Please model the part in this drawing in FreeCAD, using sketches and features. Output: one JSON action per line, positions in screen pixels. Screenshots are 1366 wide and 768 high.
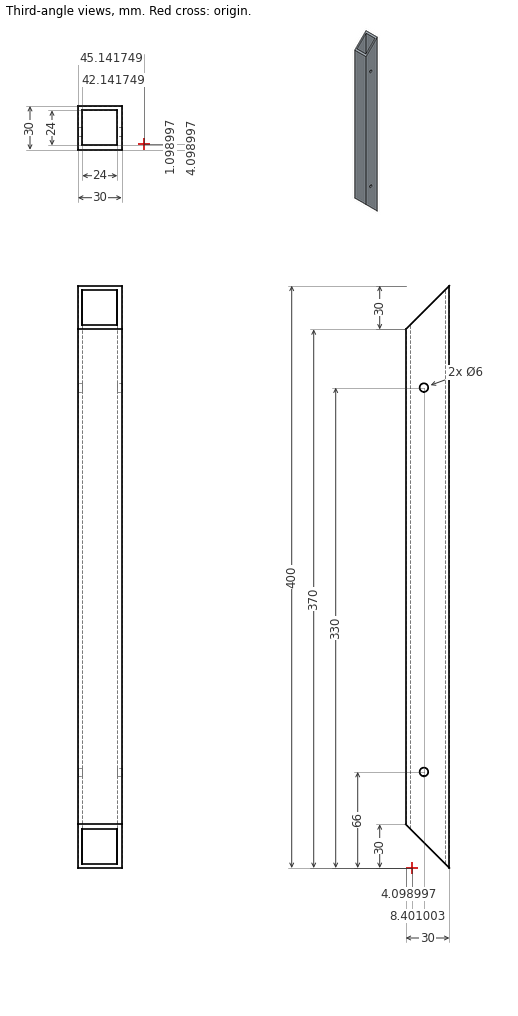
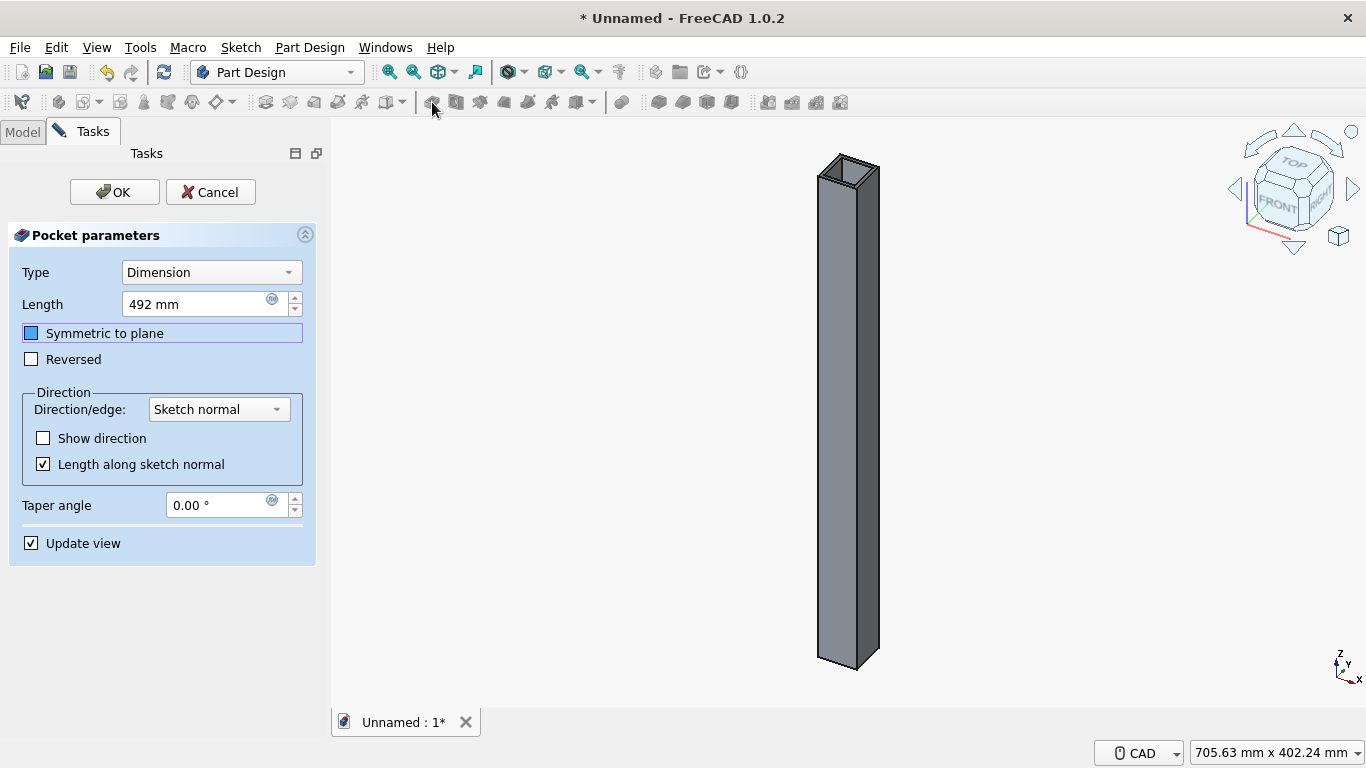
{"action": "left_click", "coordinate": [115, 192]}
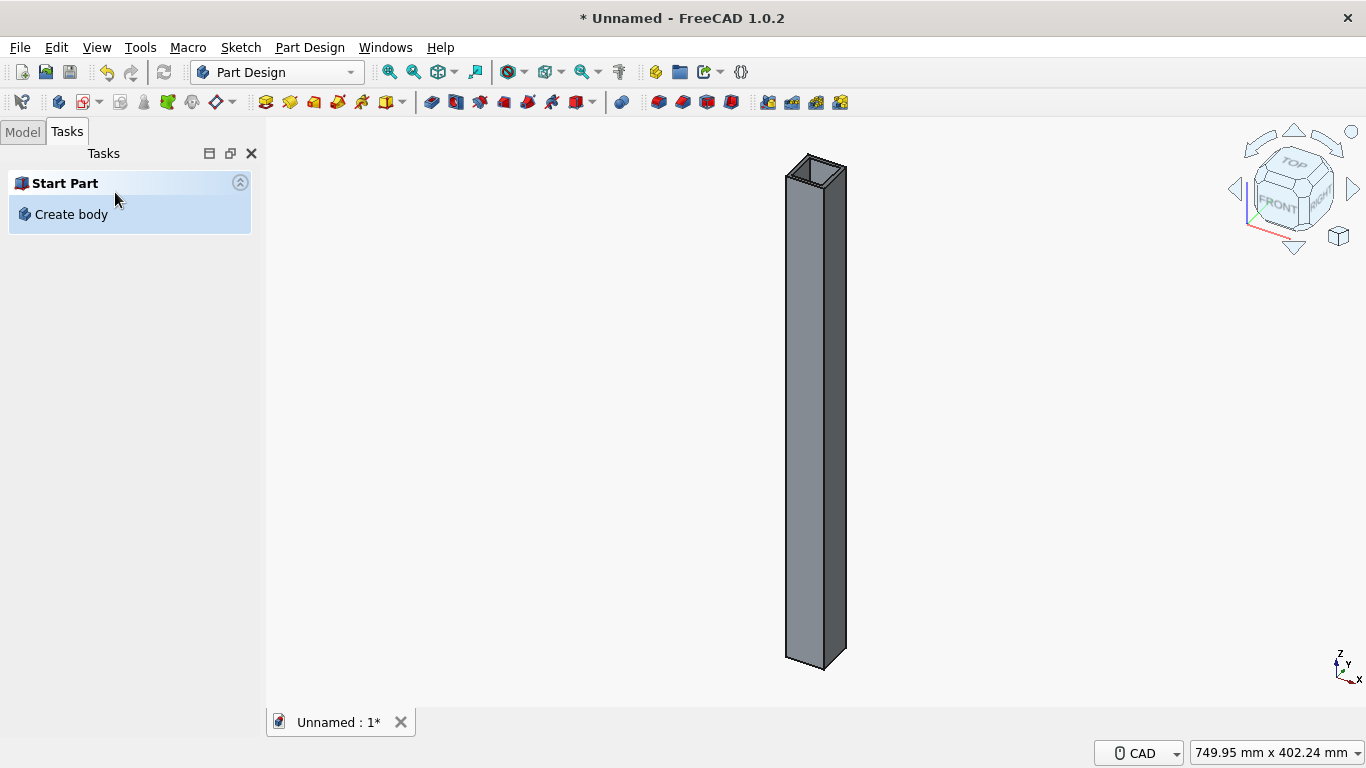
{"action": "left_click", "coordinate": [835, 211]}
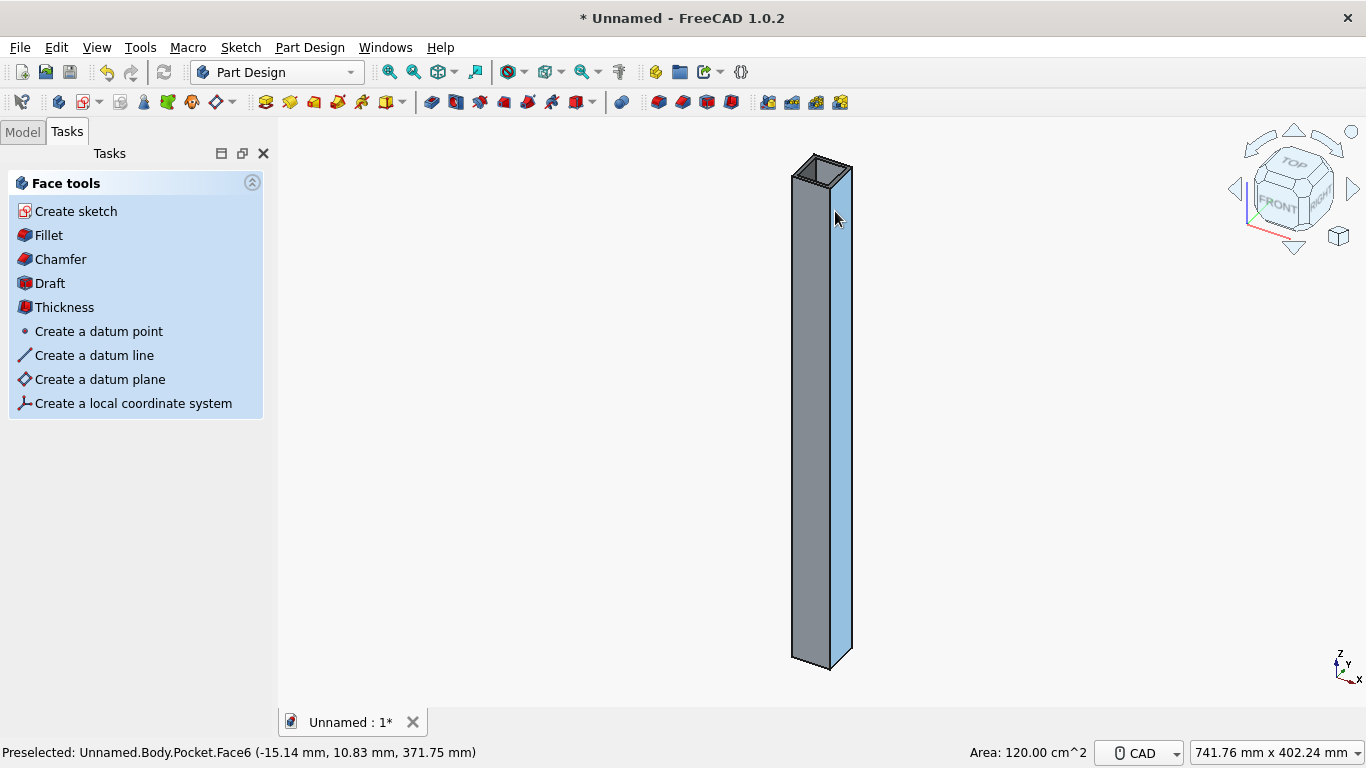
{"action": "left_click", "coordinate": [84, 102]}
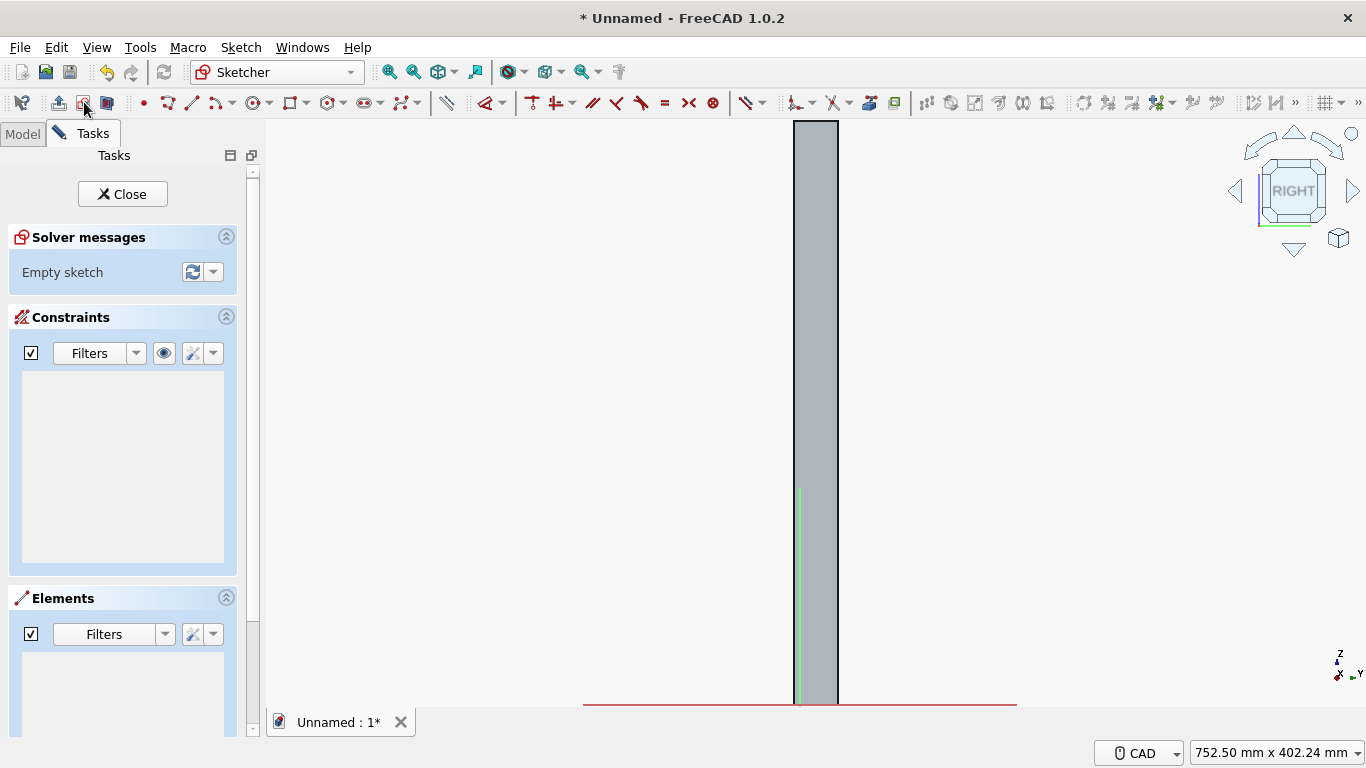
{"action": "scroll", "coordinate": [748, 413], "scroll_direction": "down", "scroll_amount": 5}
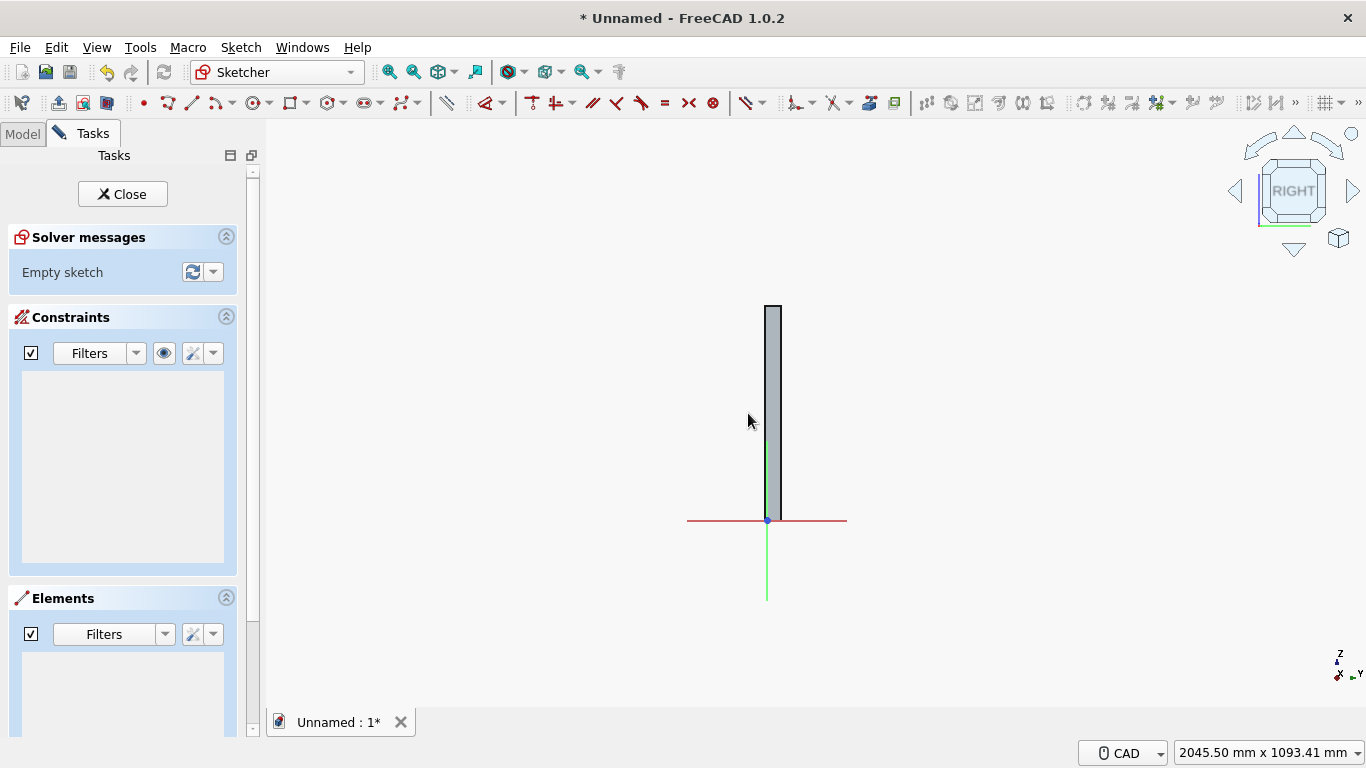
{"action": "scroll", "coordinate": [775, 518], "scroll_direction": "up", "scroll_amount": 15}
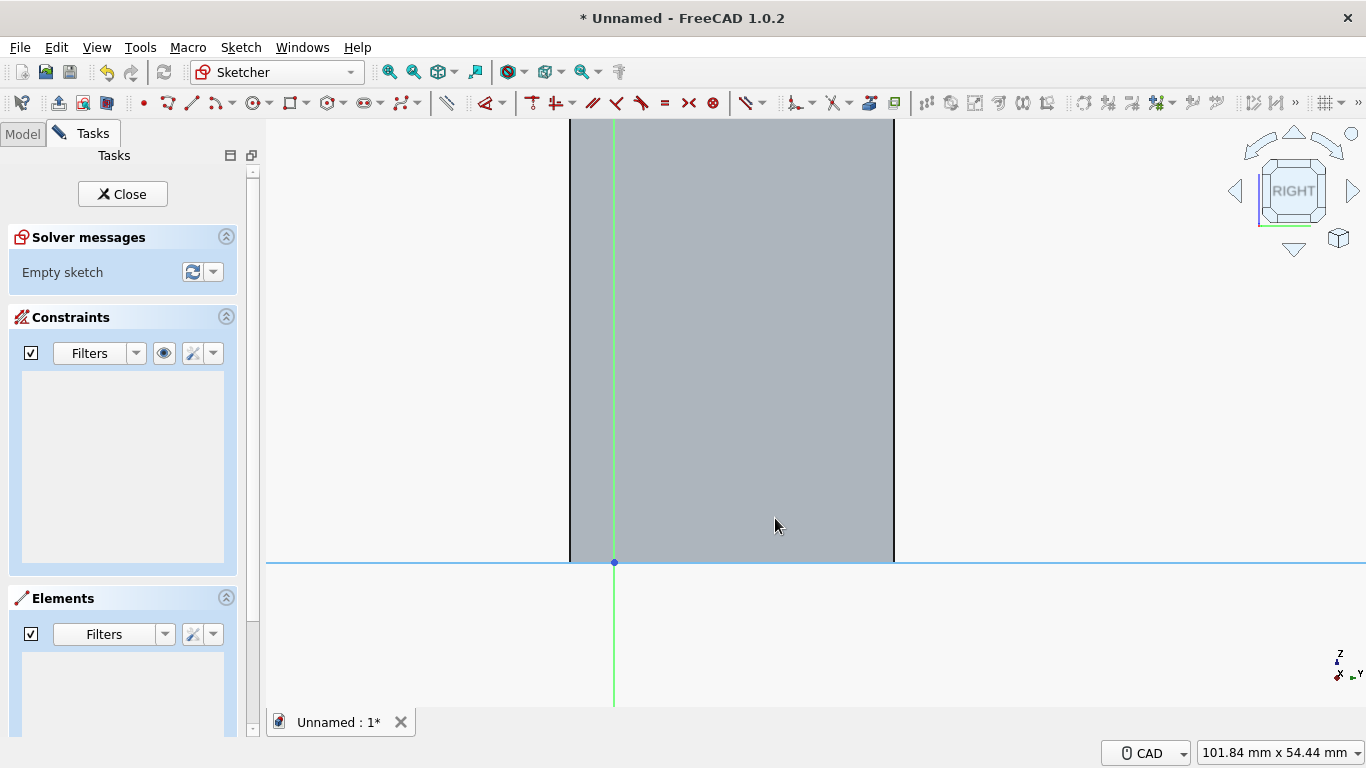
{"action": "left_click", "coordinate": [168, 104]}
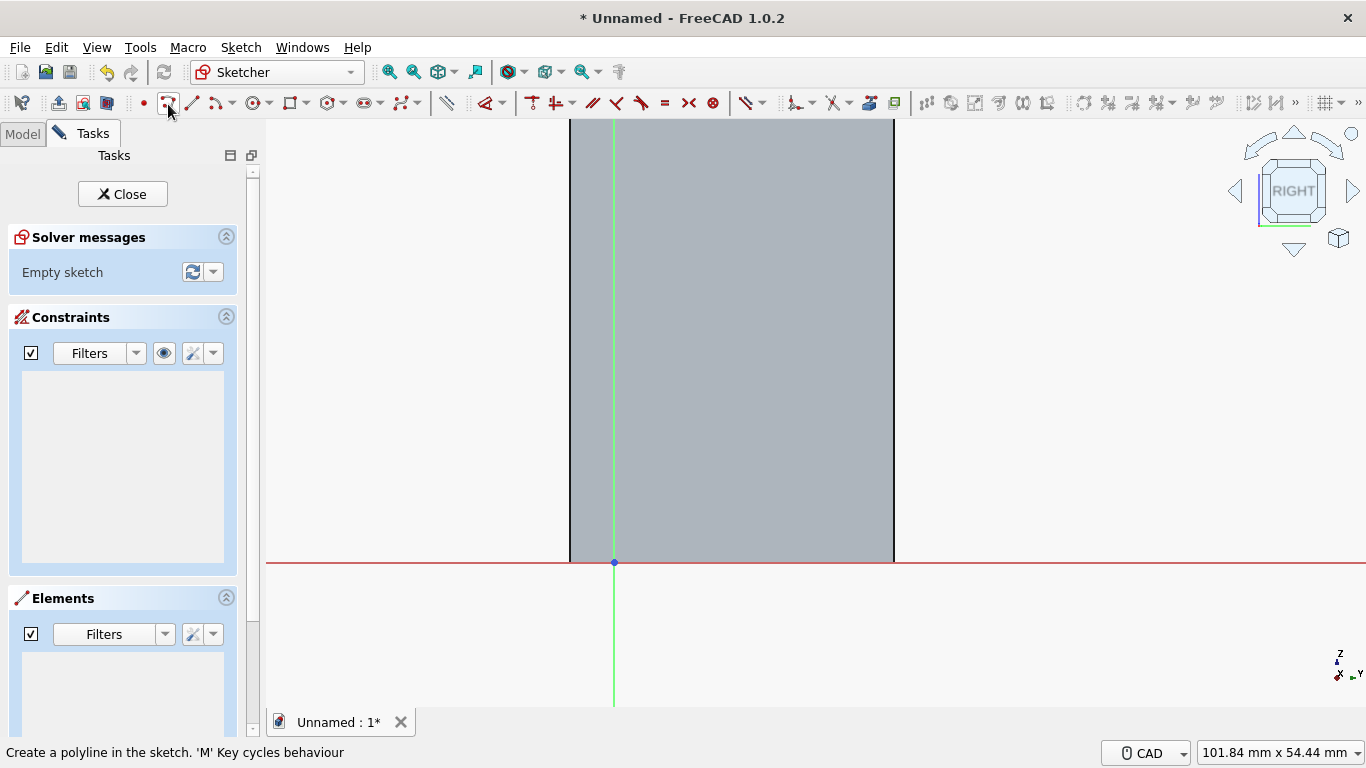
{"action": "left_click", "coordinate": [570, 563]}
{"action": "left_click", "coordinate": [894, 554]}
{"action": "left_click", "coordinate": [570, 239]}
{"action": "left_click", "coordinate": [570, 563]}
{"action": "key", "text": "Escape"}
{"action": "key", "text": "Escape"}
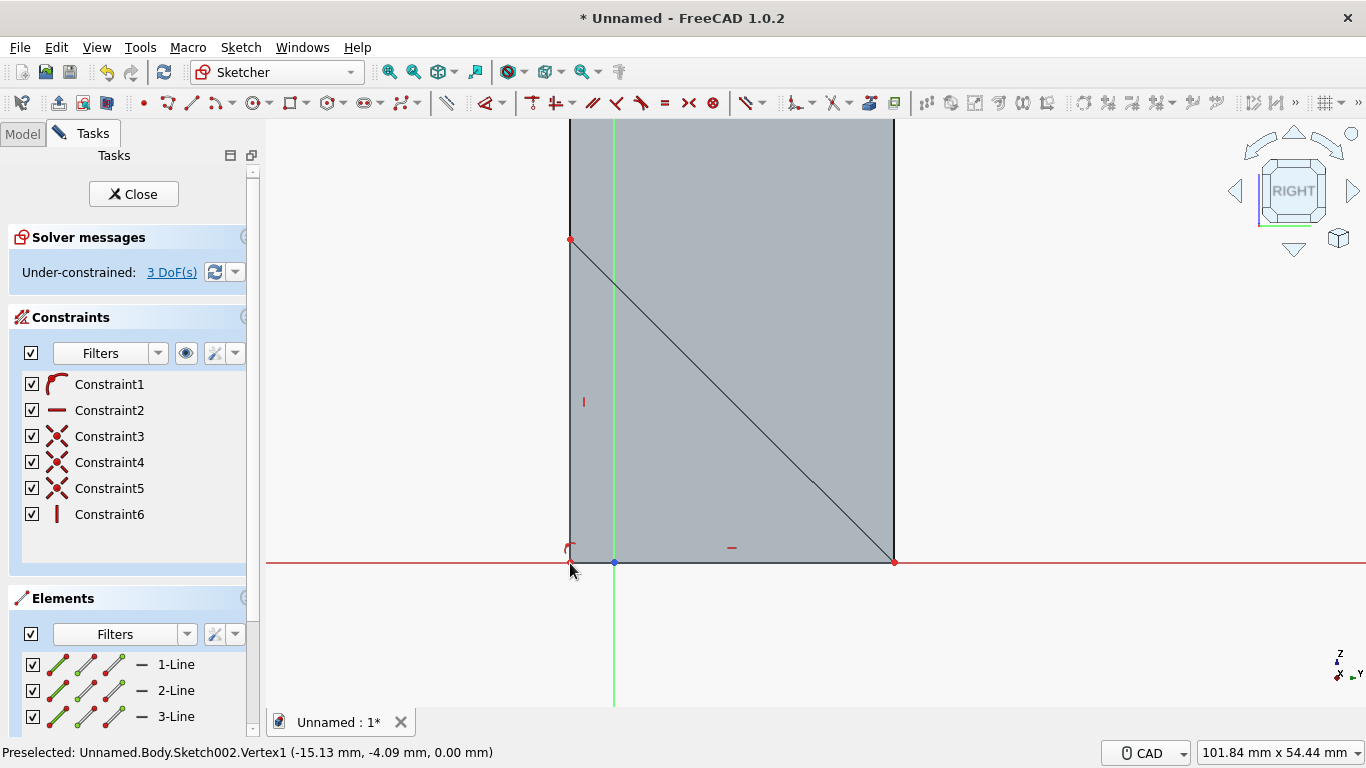
{"action": "key", "text": "d"}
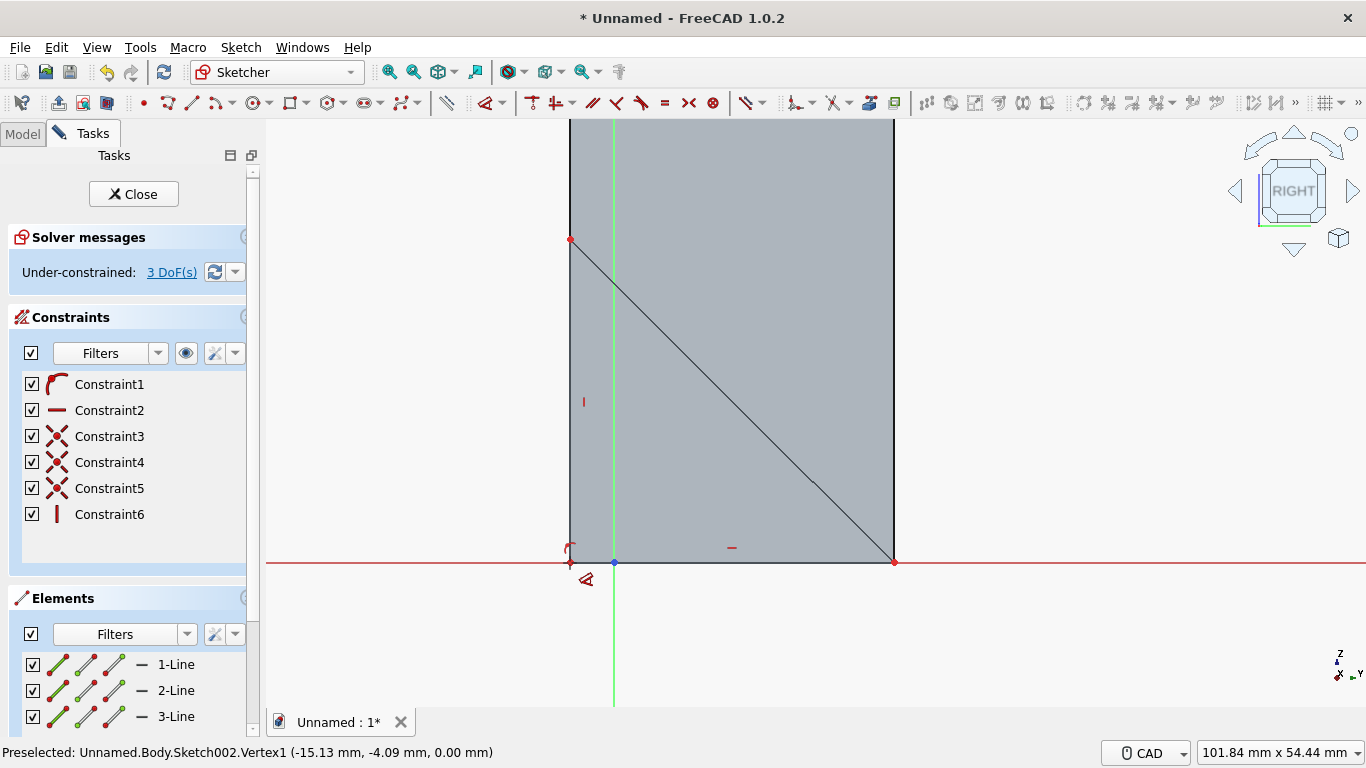
{"action": "left_click", "coordinate": [667, 563]}
{"action": "left_click", "coordinate": [732, 597]}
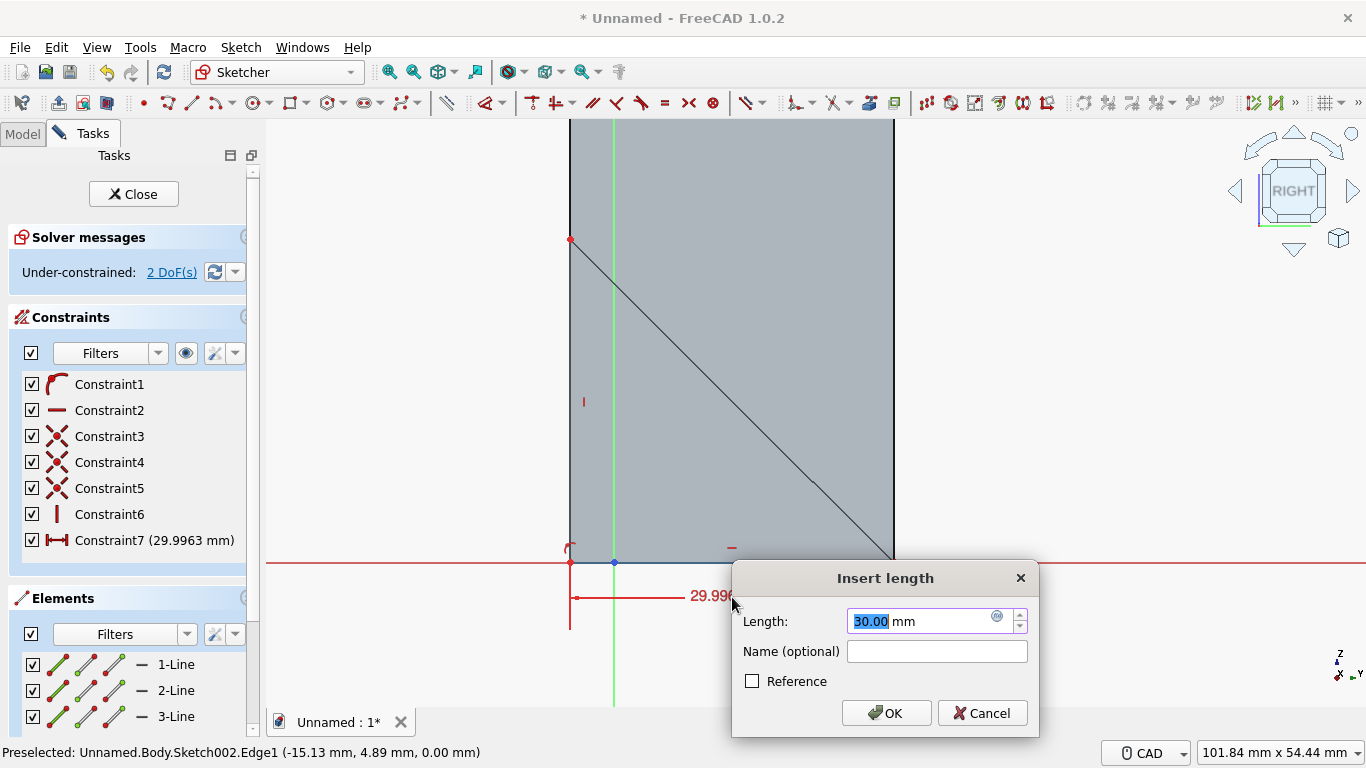
{"action": "type", "text": "30"}
{"action": "key", "text": "Return"}